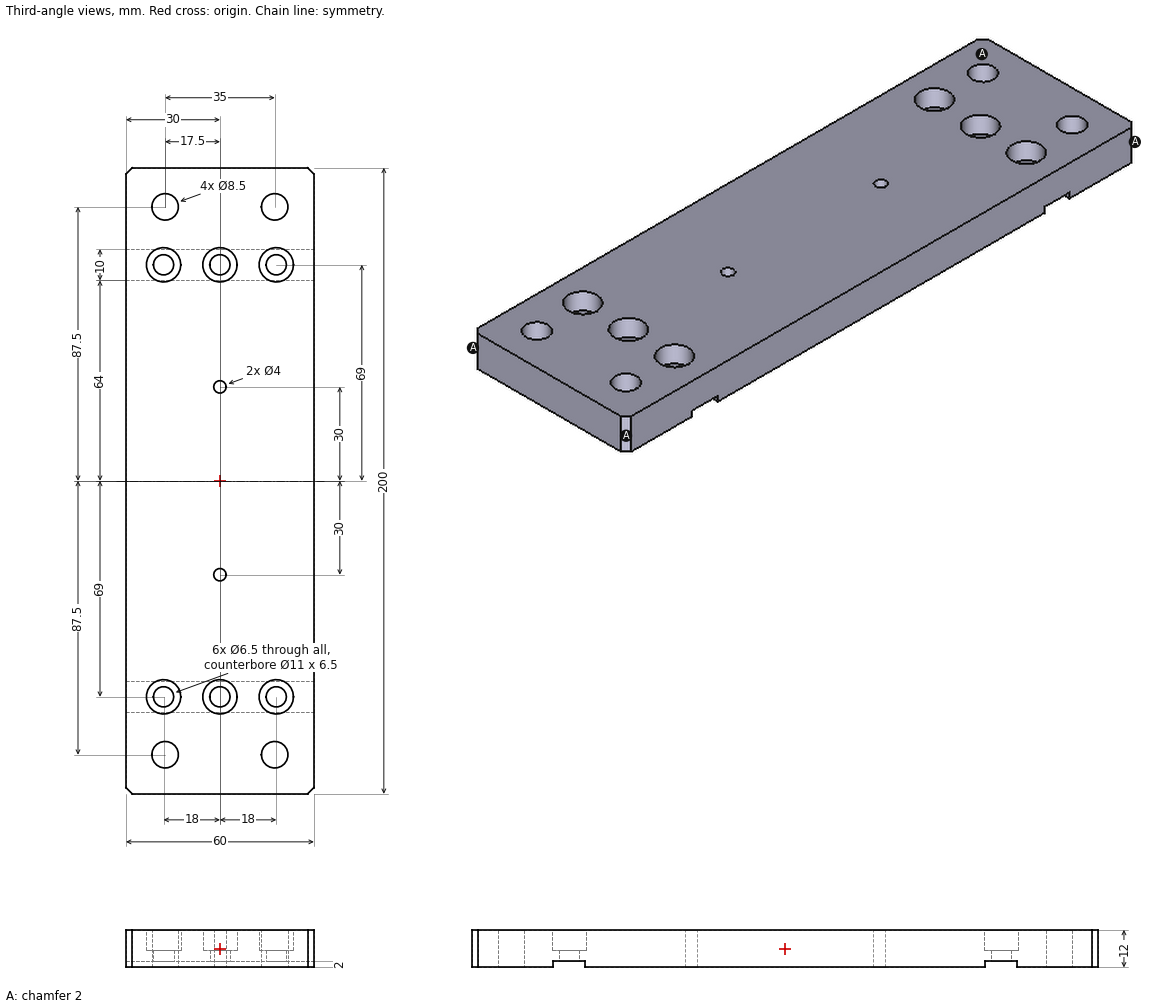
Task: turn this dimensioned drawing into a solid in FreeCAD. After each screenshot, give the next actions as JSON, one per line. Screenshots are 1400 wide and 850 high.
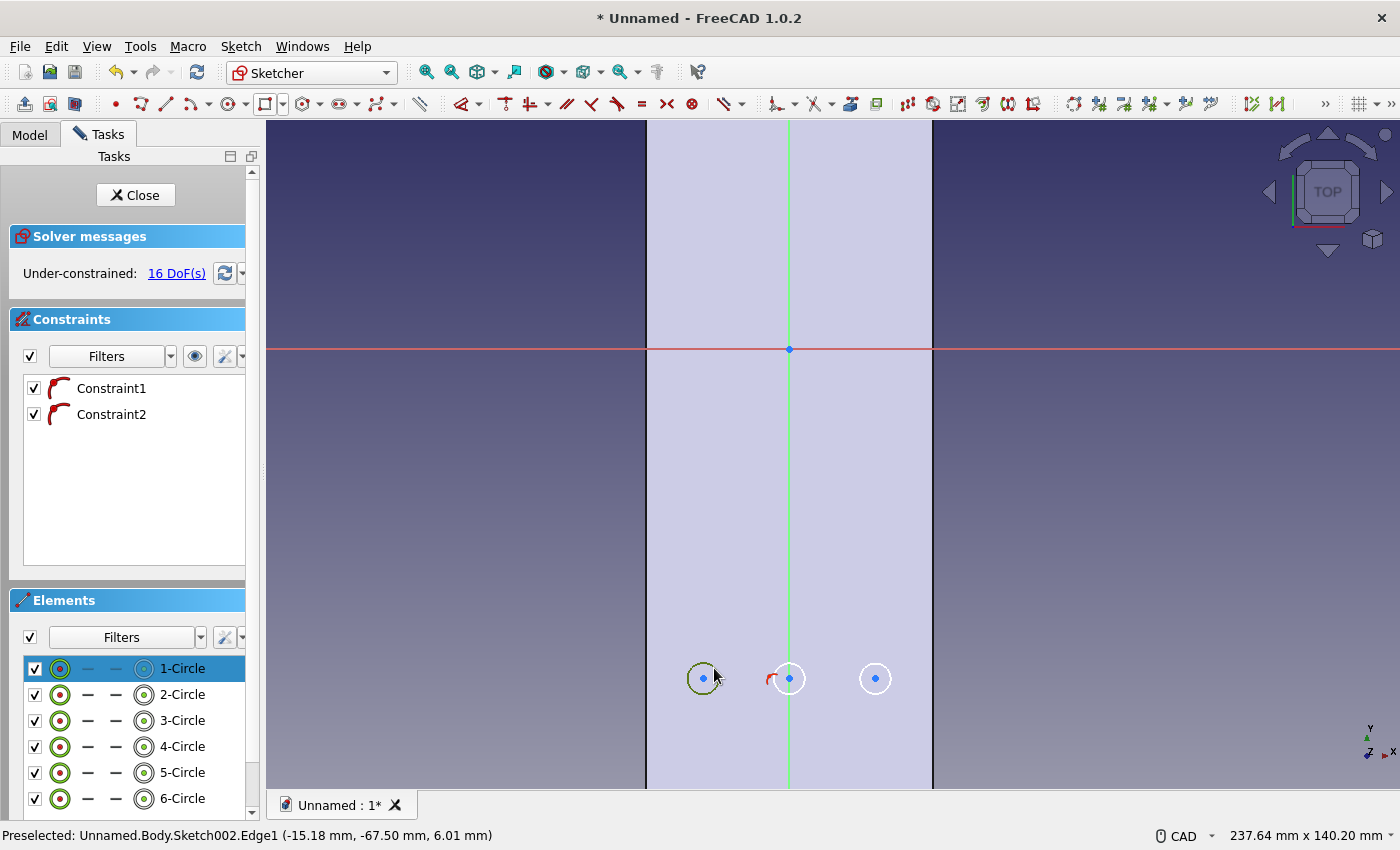
{"action": "scroll", "coordinate": [800, 668], "scroll_direction": "up", "scroll_amount": 2}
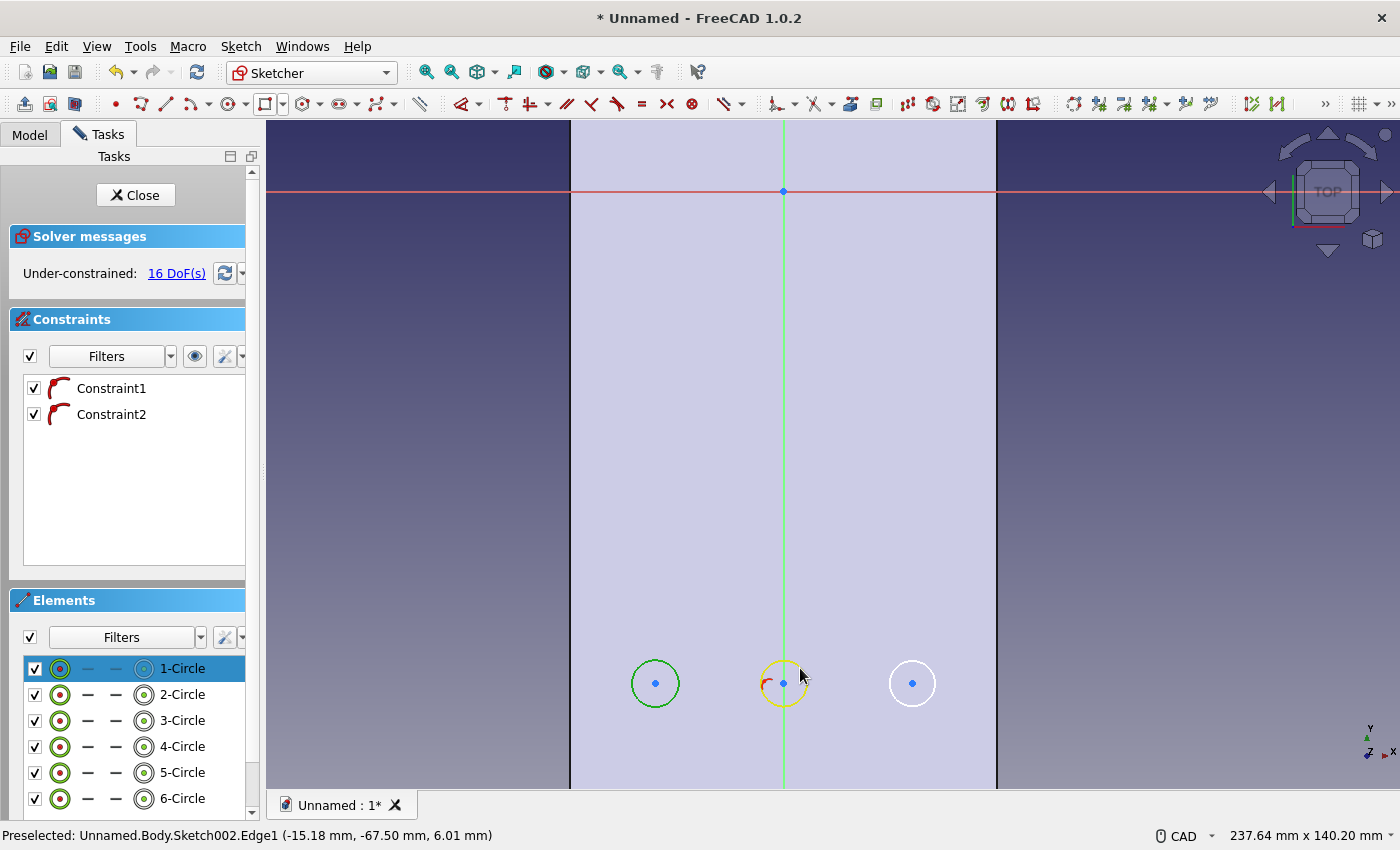
{"action": "left_click", "coordinate": [800, 667]}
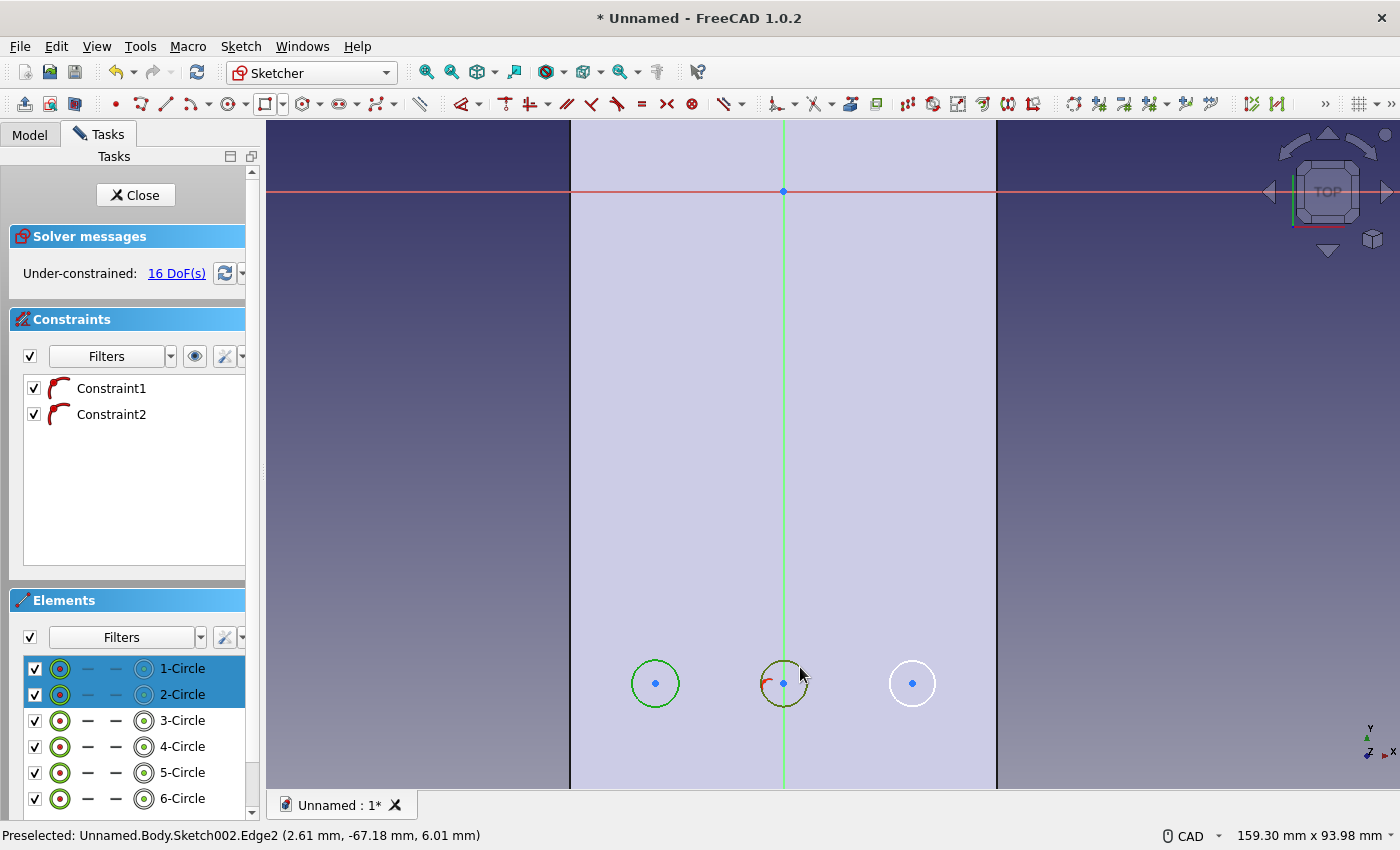
{"action": "left_click", "coordinate": [928, 668]}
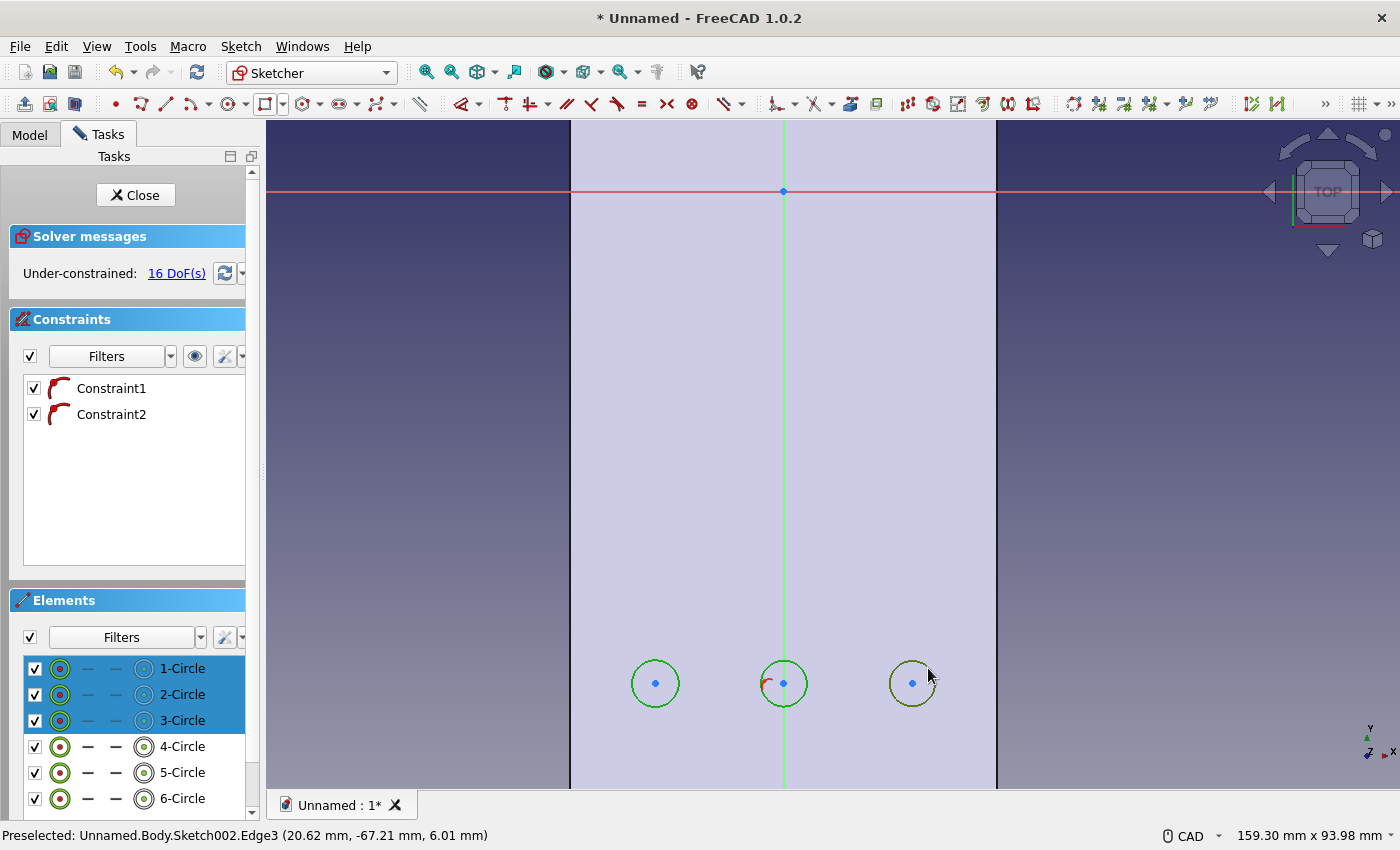
{"action": "scroll", "coordinate": [749, 669], "scroll_direction": "down", "scroll_amount": 4}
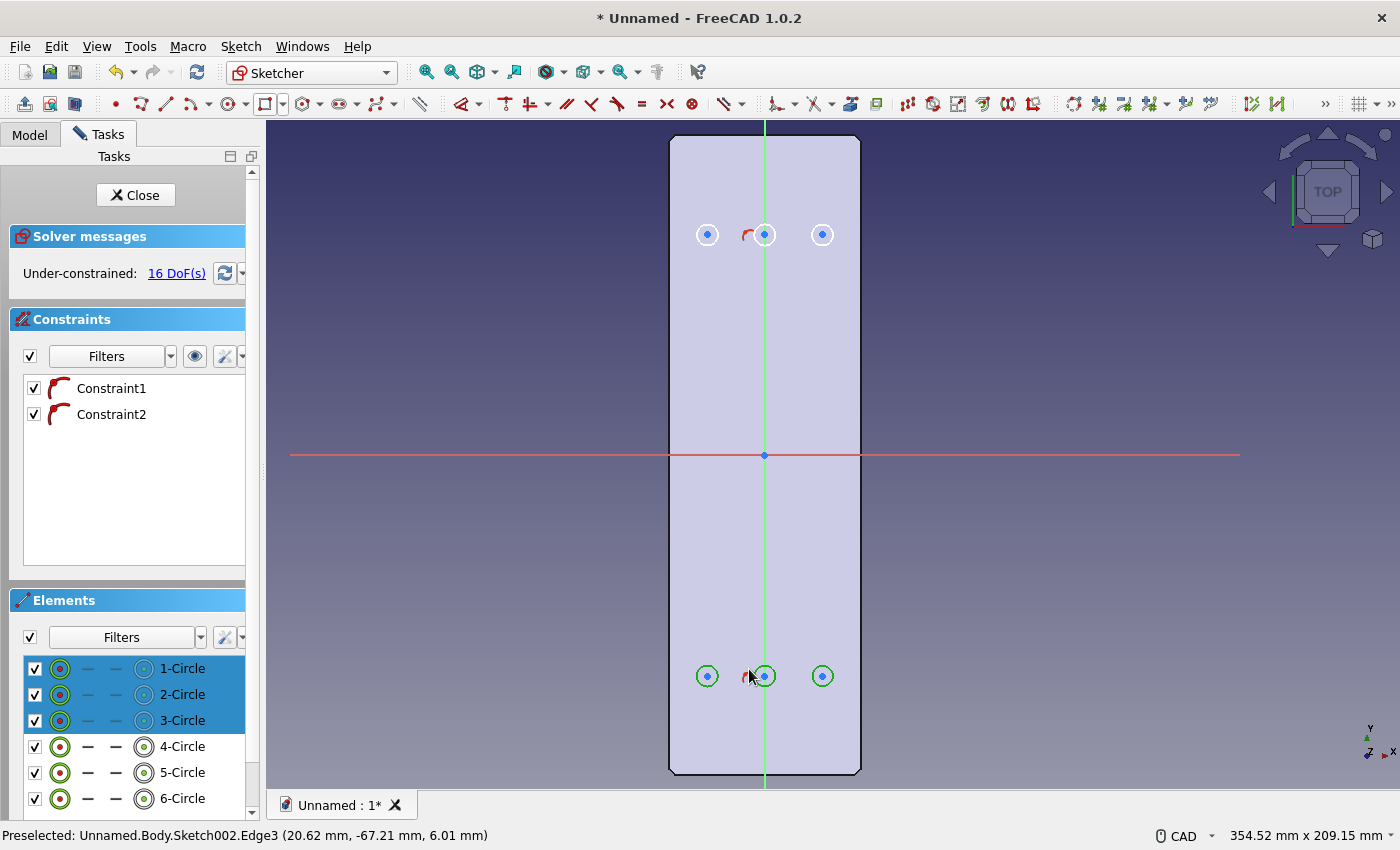
{"action": "scroll", "coordinate": [830, 228], "scroll_direction": "up", "scroll_amount": 2}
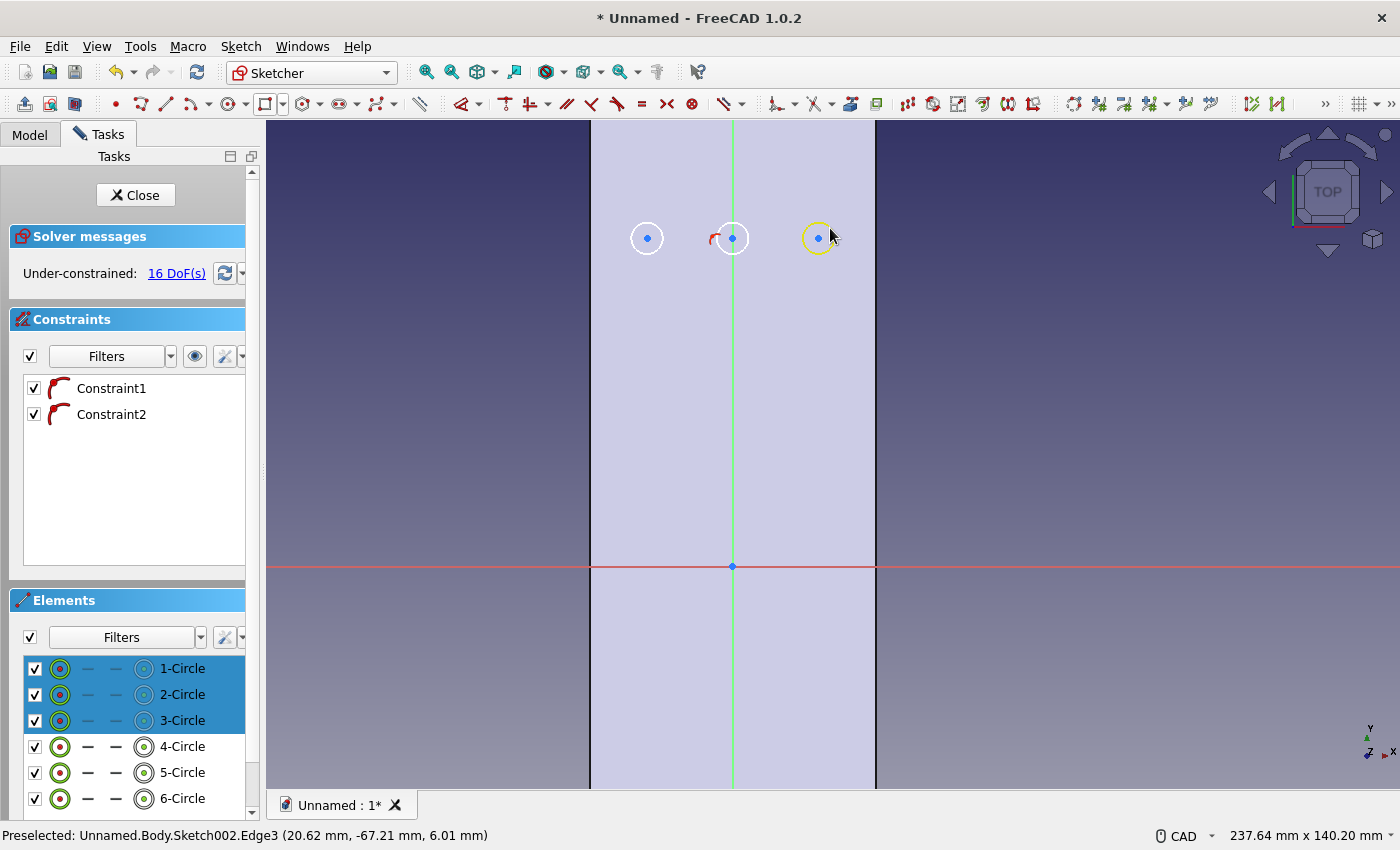
{"action": "left_click", "coordinate": [830, 227]}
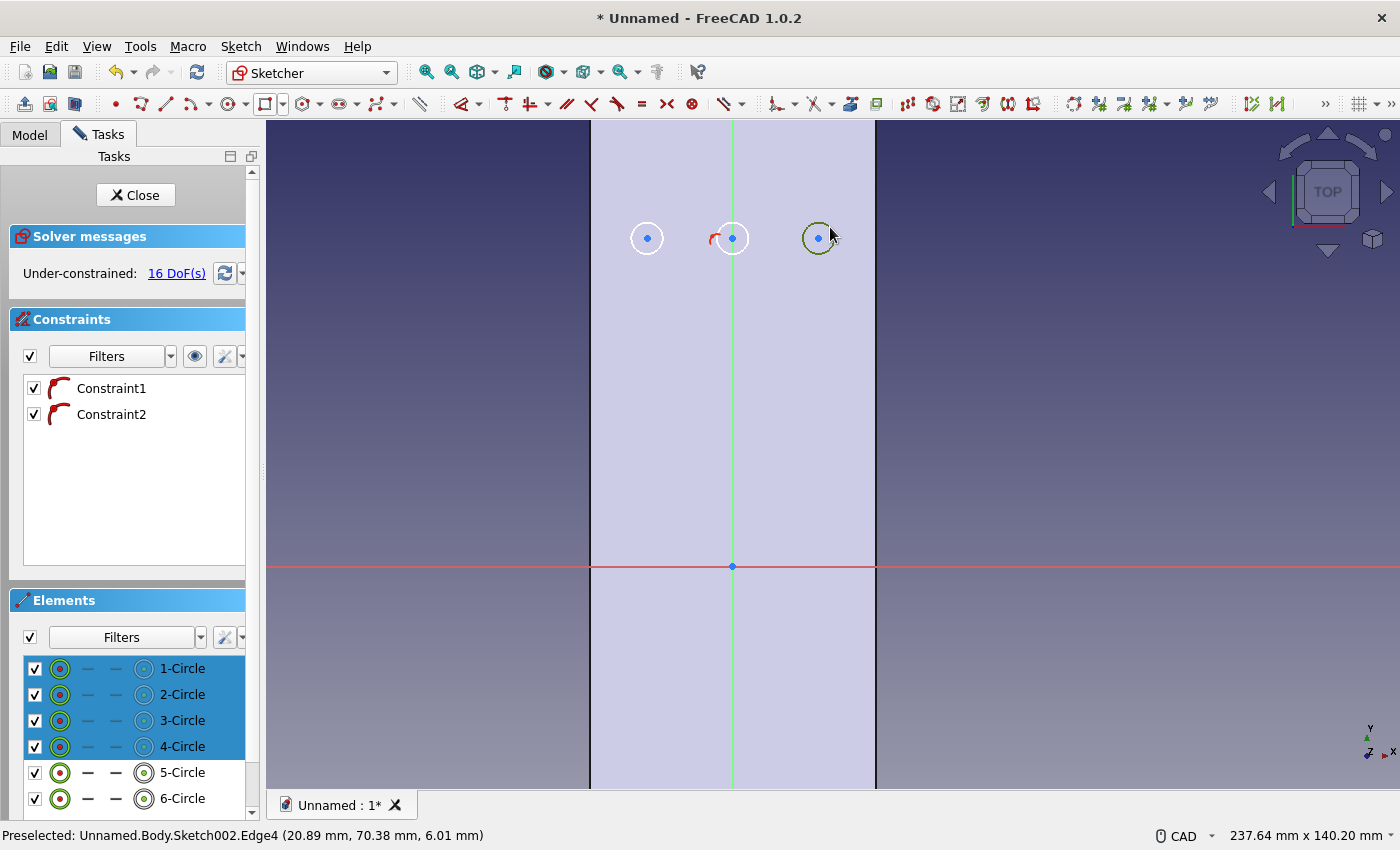
{"action": "scroll", "coordinate": [744, 227], "scroll_direction": "up", "scroll_amount": 2}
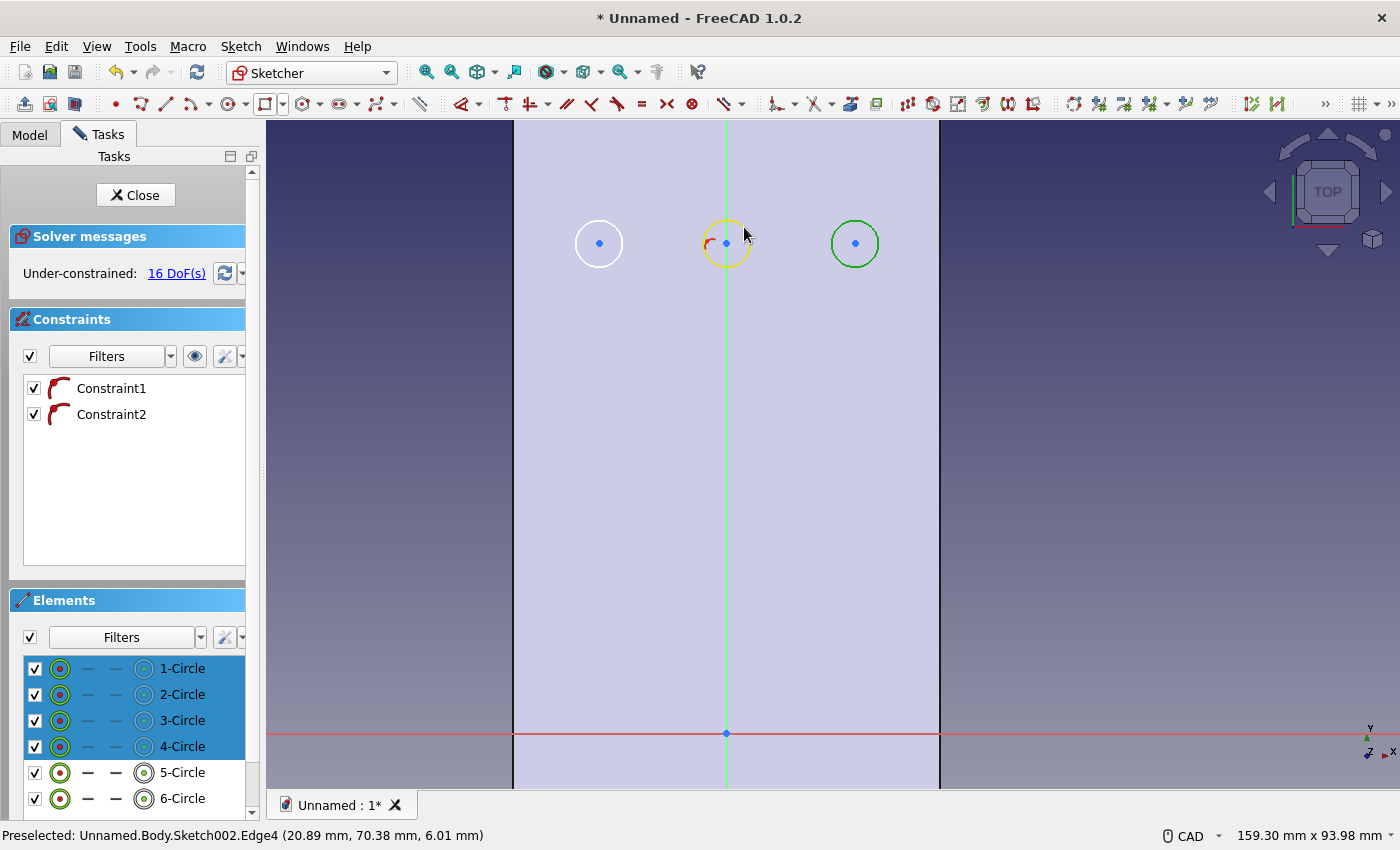
{"action": "left_click", "coordinate": [743, 227]}